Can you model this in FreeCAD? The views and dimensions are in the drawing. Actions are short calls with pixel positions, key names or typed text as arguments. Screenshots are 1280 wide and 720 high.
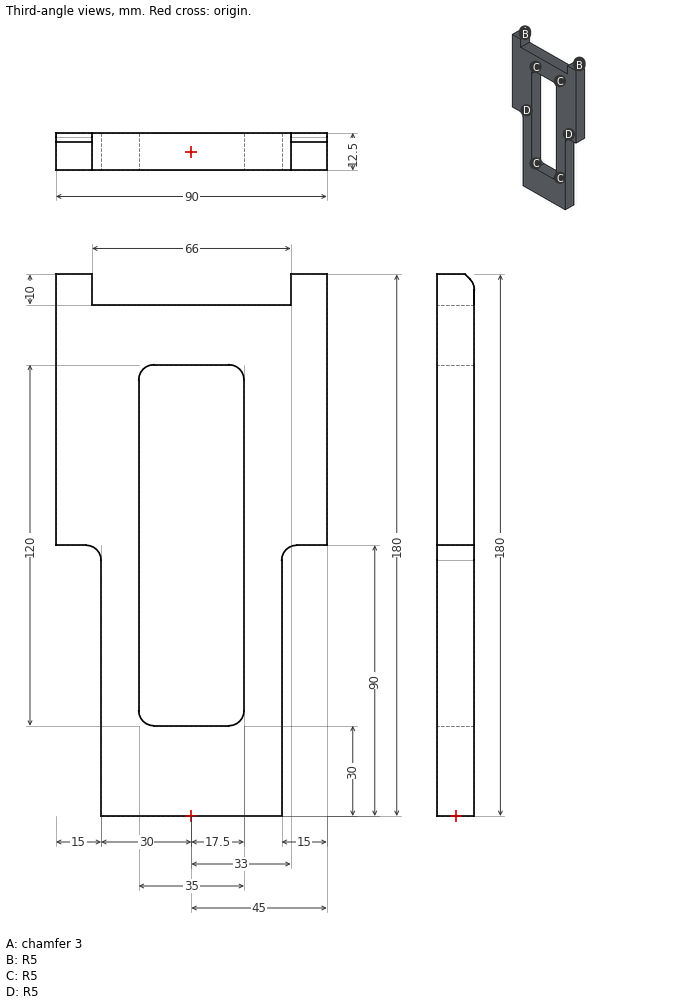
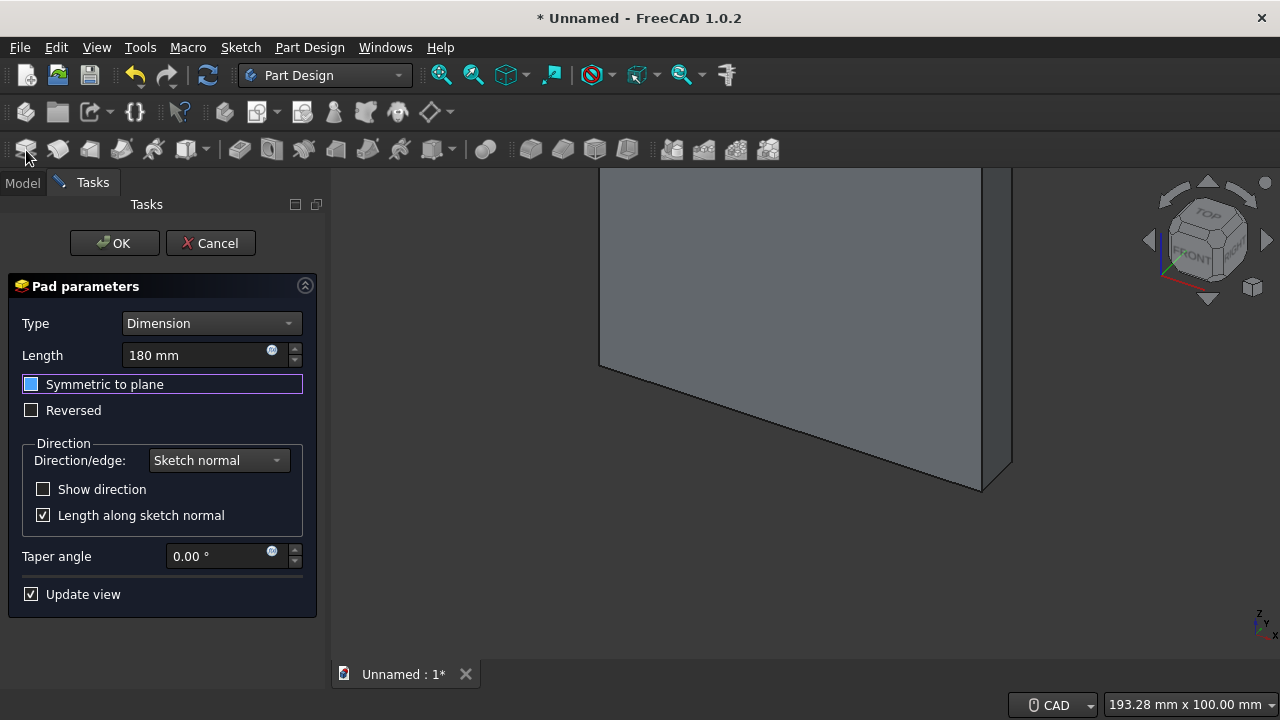
click(115, 243)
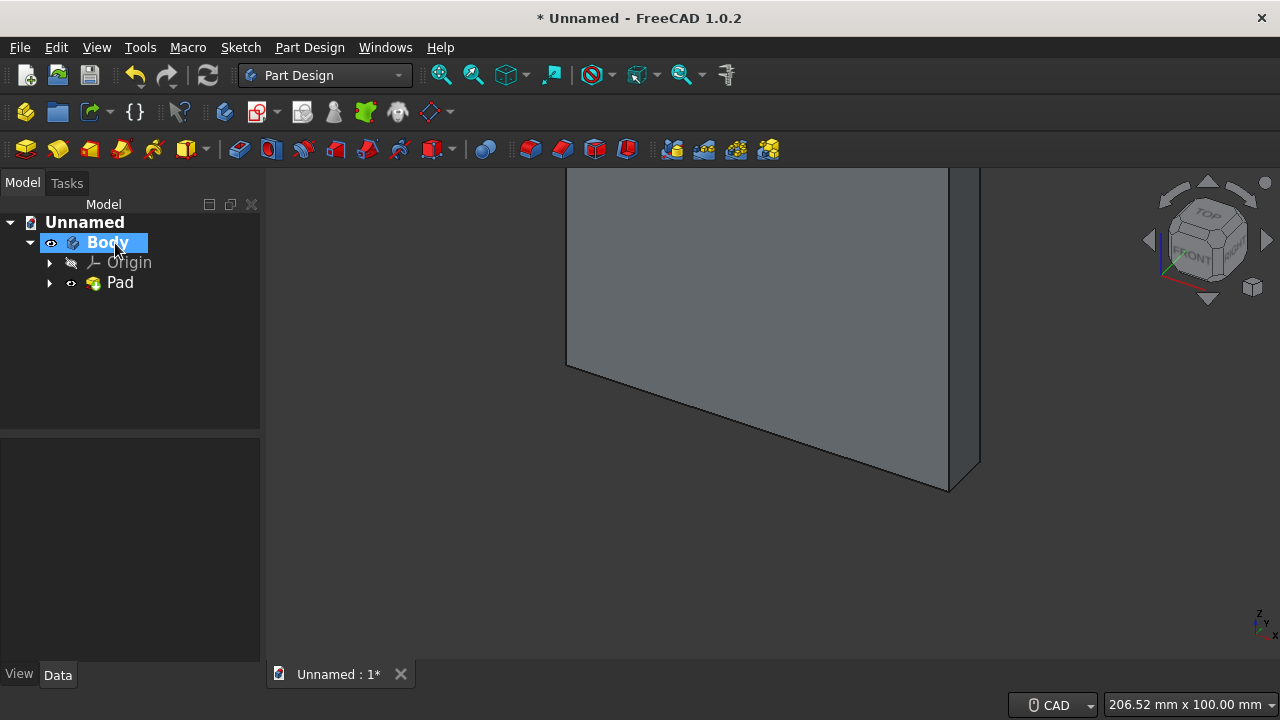
click(442, 76)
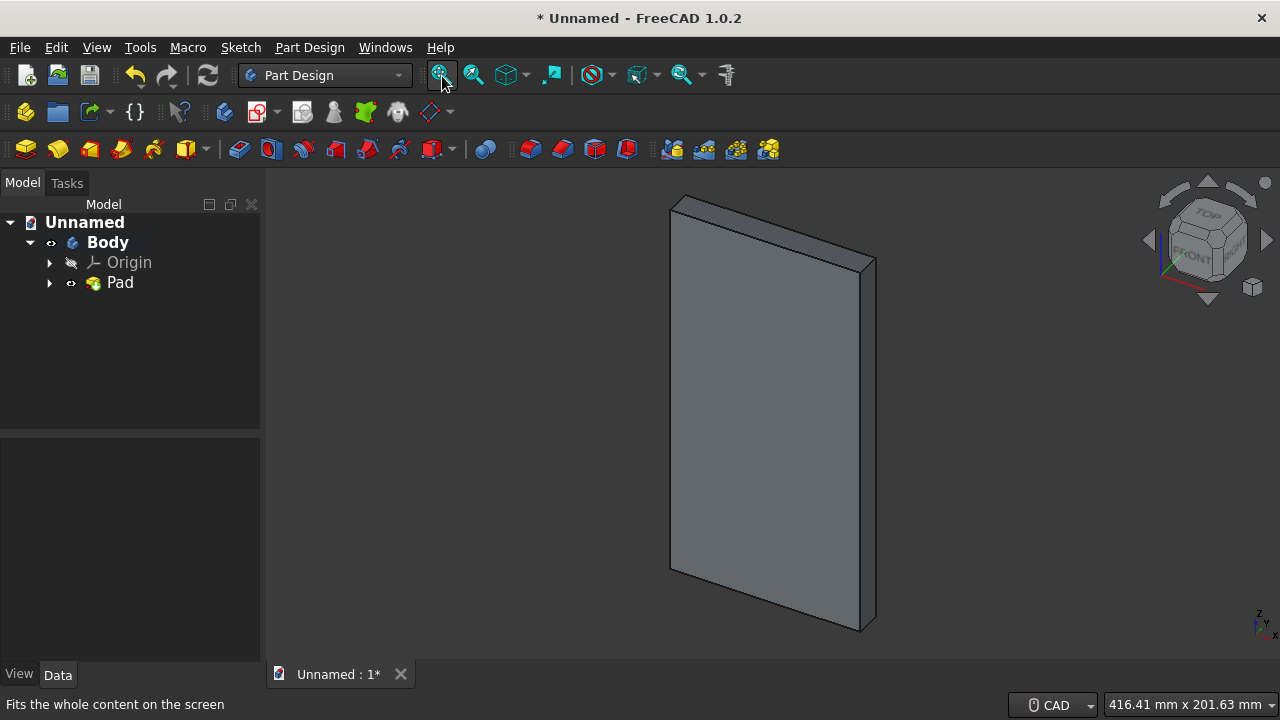
key(4)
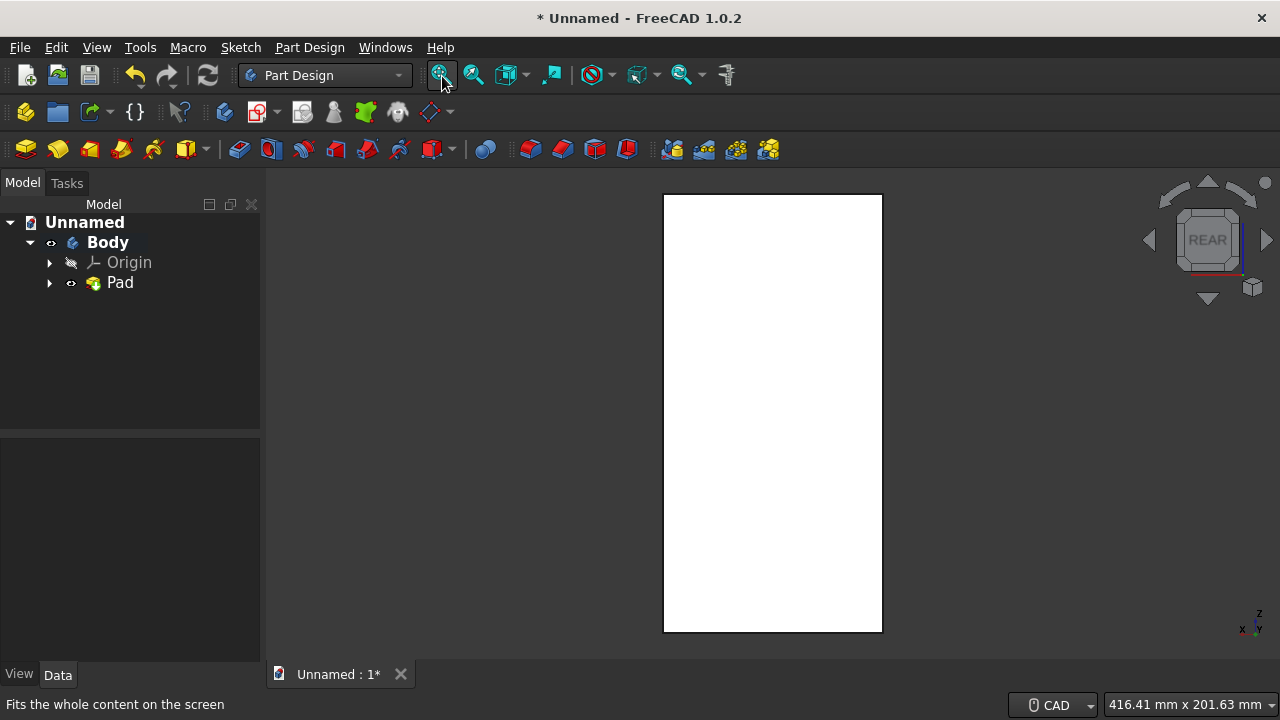
click(773, 350)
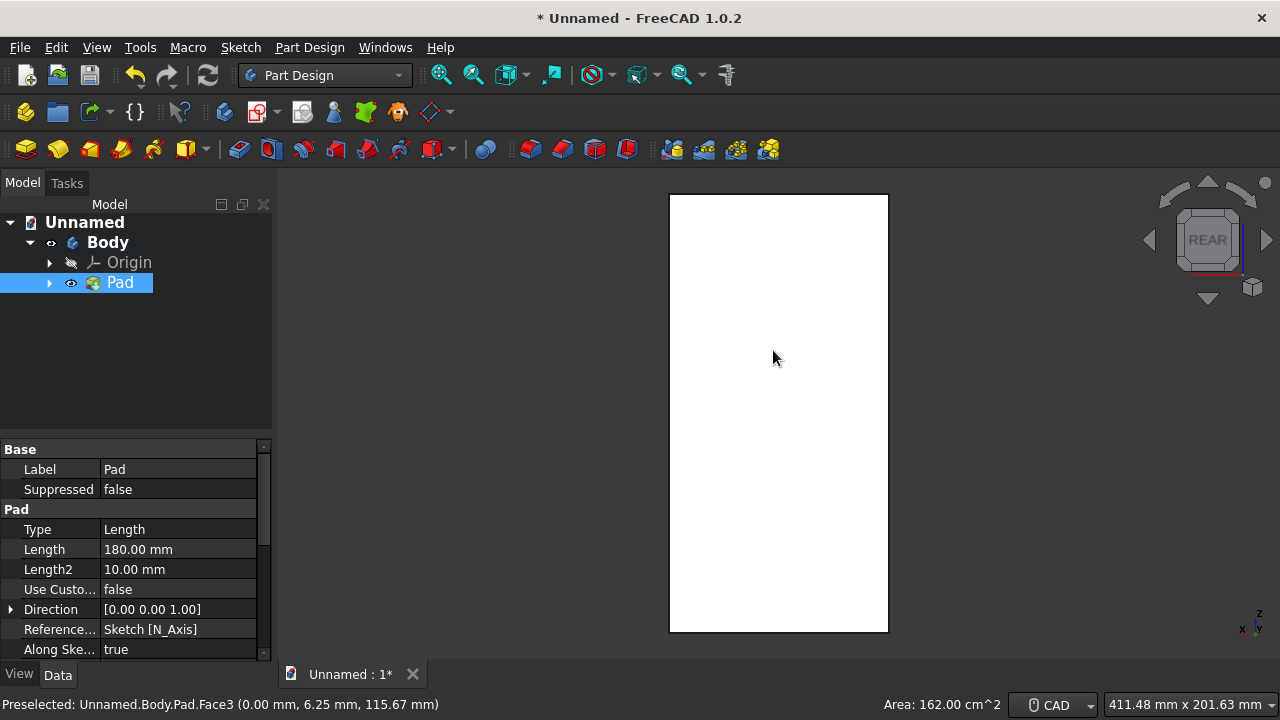
click(258, 112)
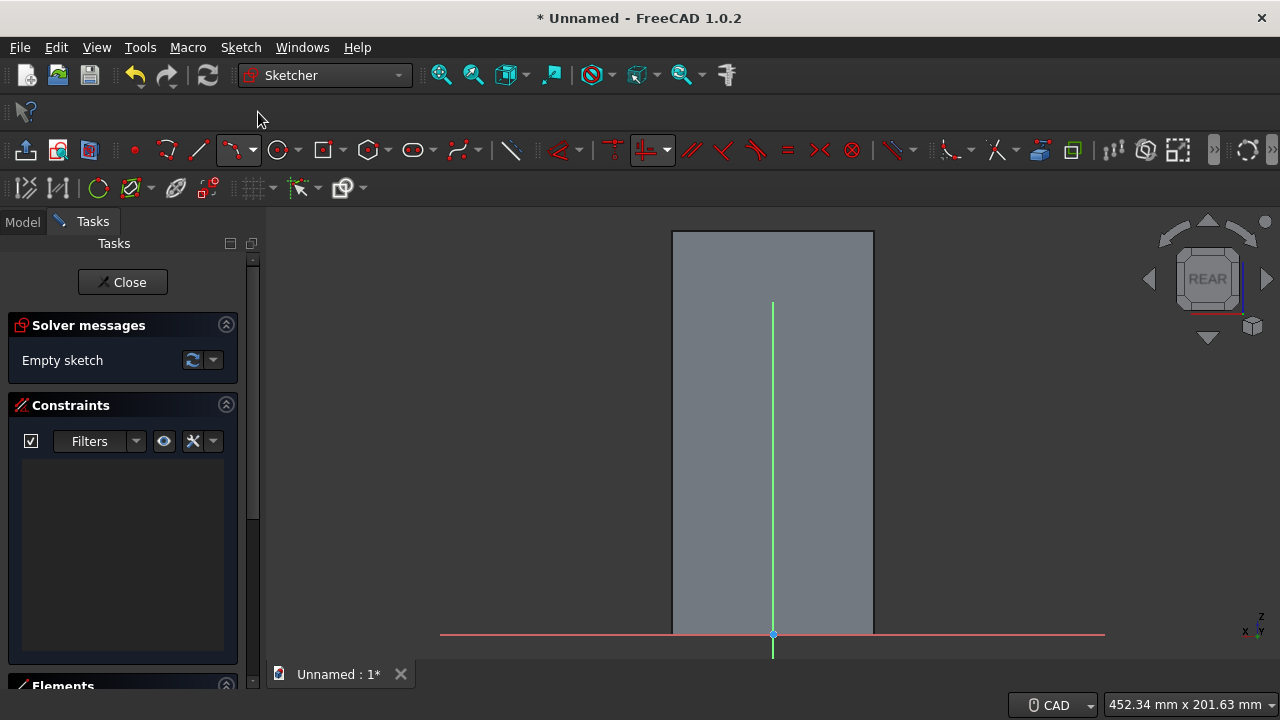
scroll(704, 433, down, 5)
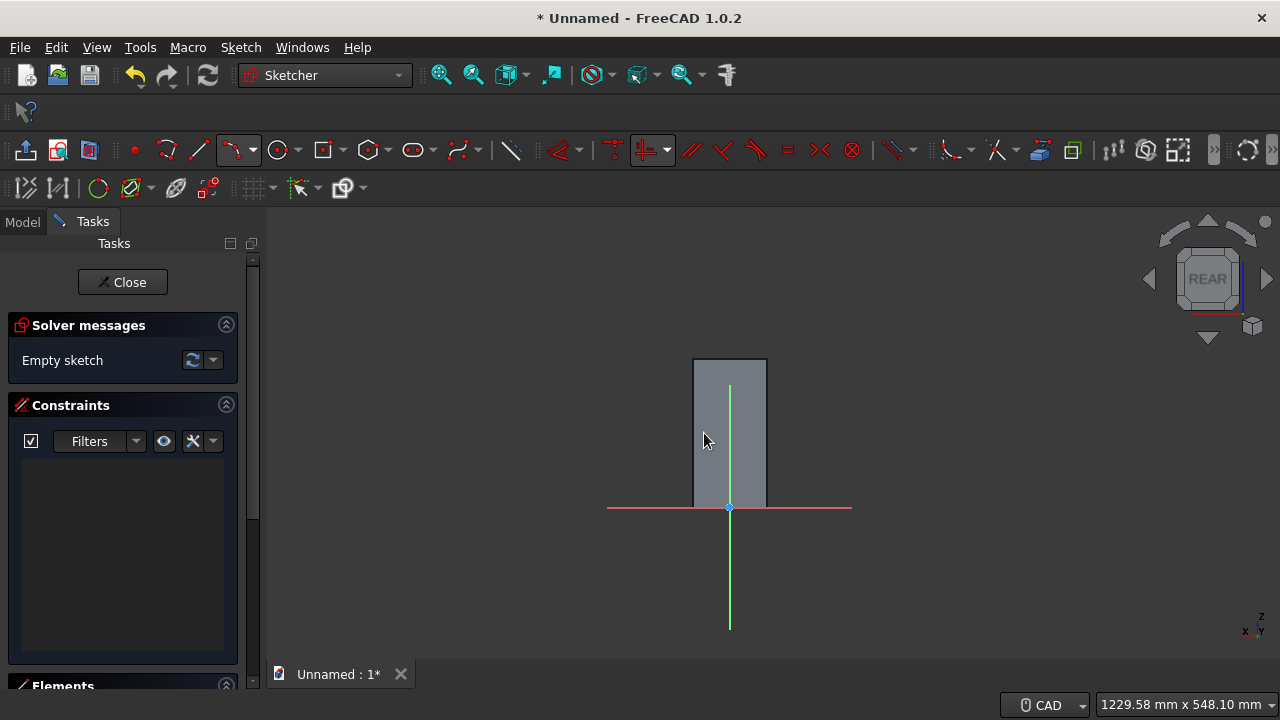
scroll(732, 356, up, 12)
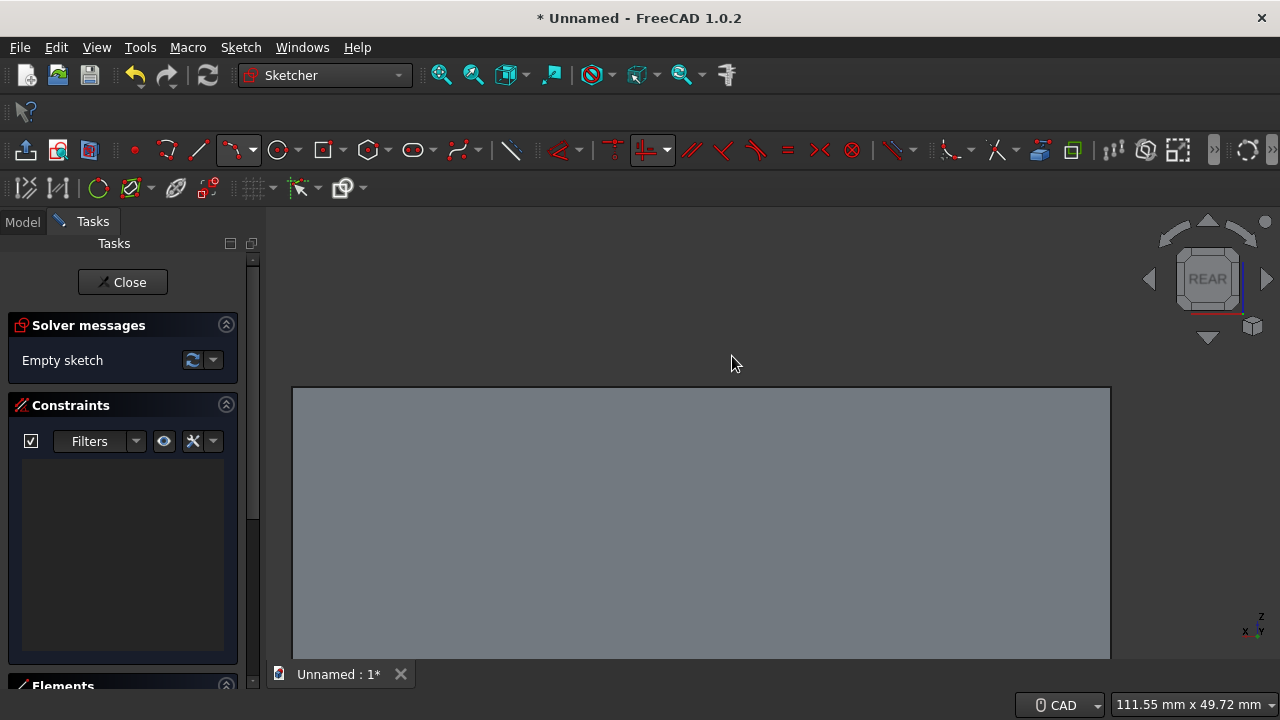
key(g)
key(r)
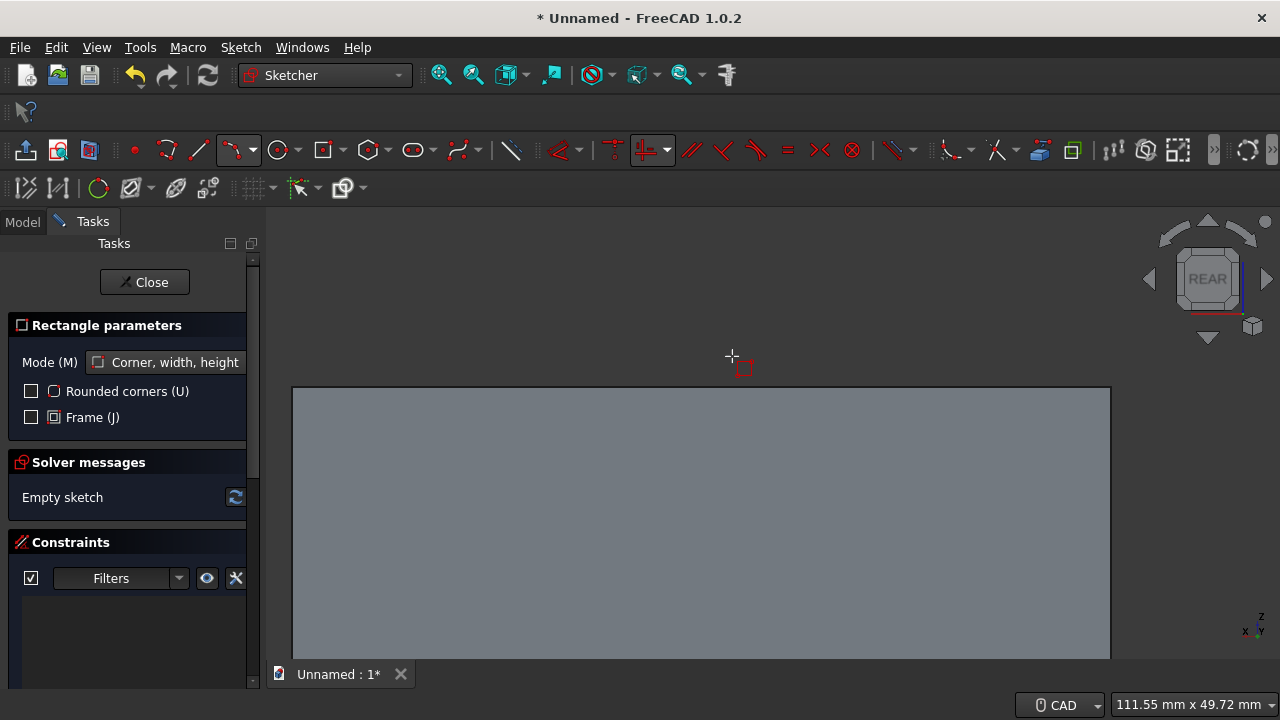
click(402, 387)
move(1002, 478)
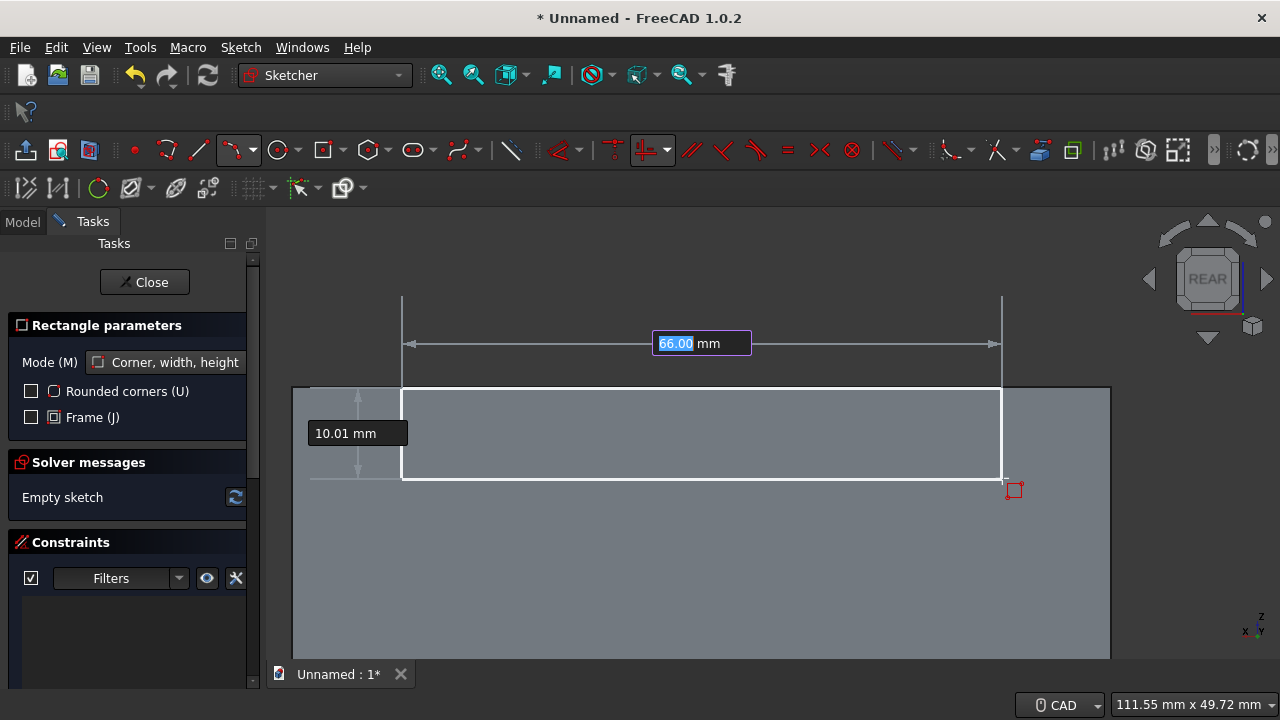
text(66)
key(Tab)
text(10)
key(Return)
key(Escape)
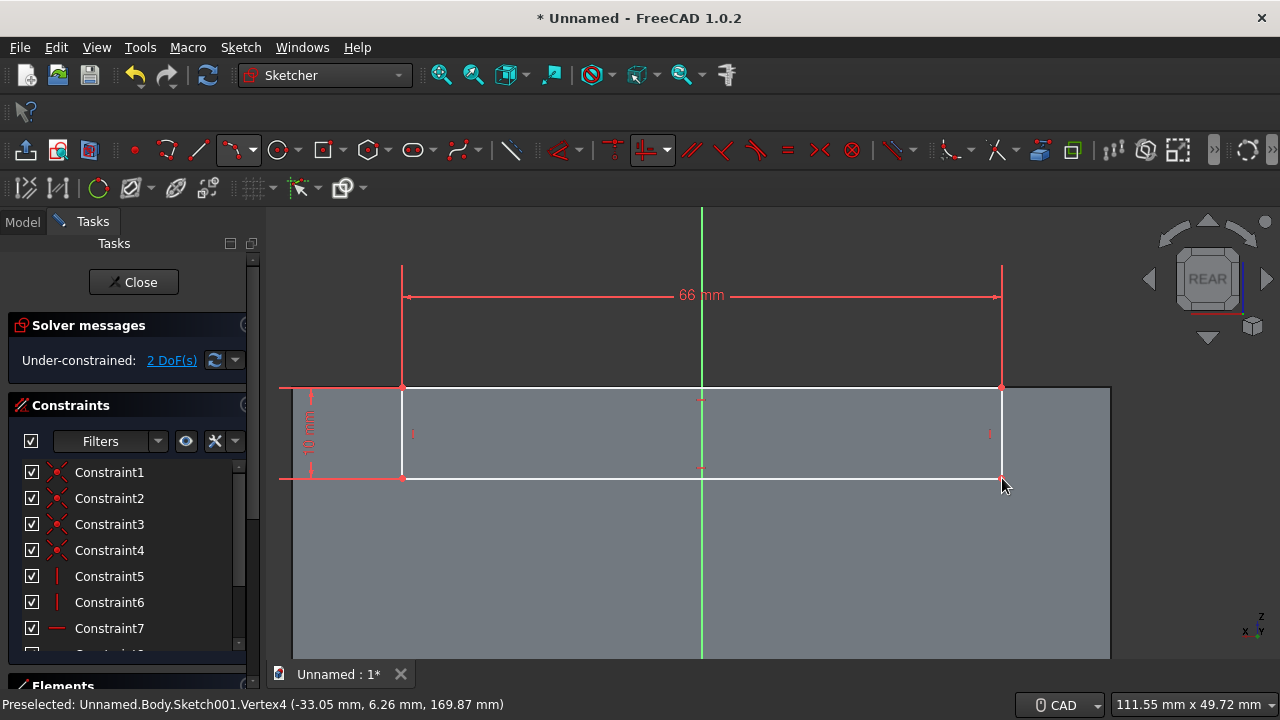
click(402, 388)